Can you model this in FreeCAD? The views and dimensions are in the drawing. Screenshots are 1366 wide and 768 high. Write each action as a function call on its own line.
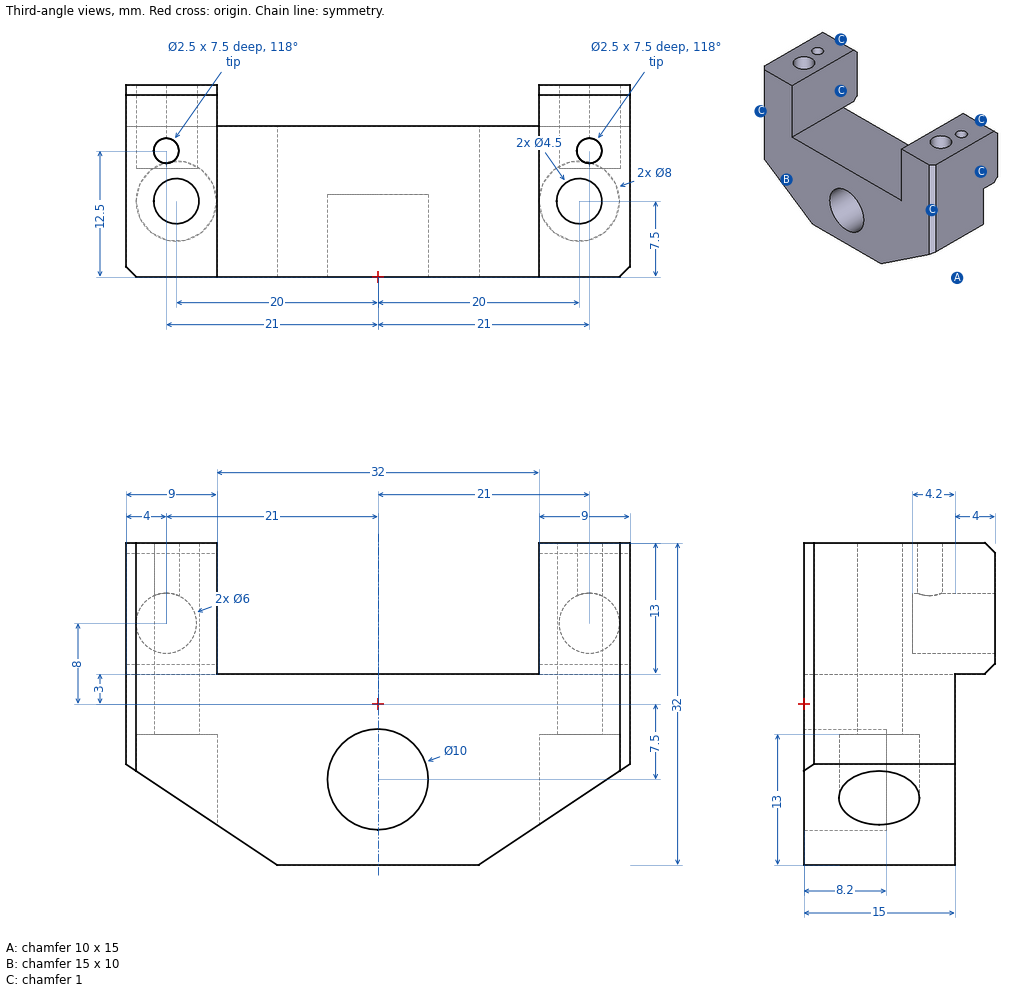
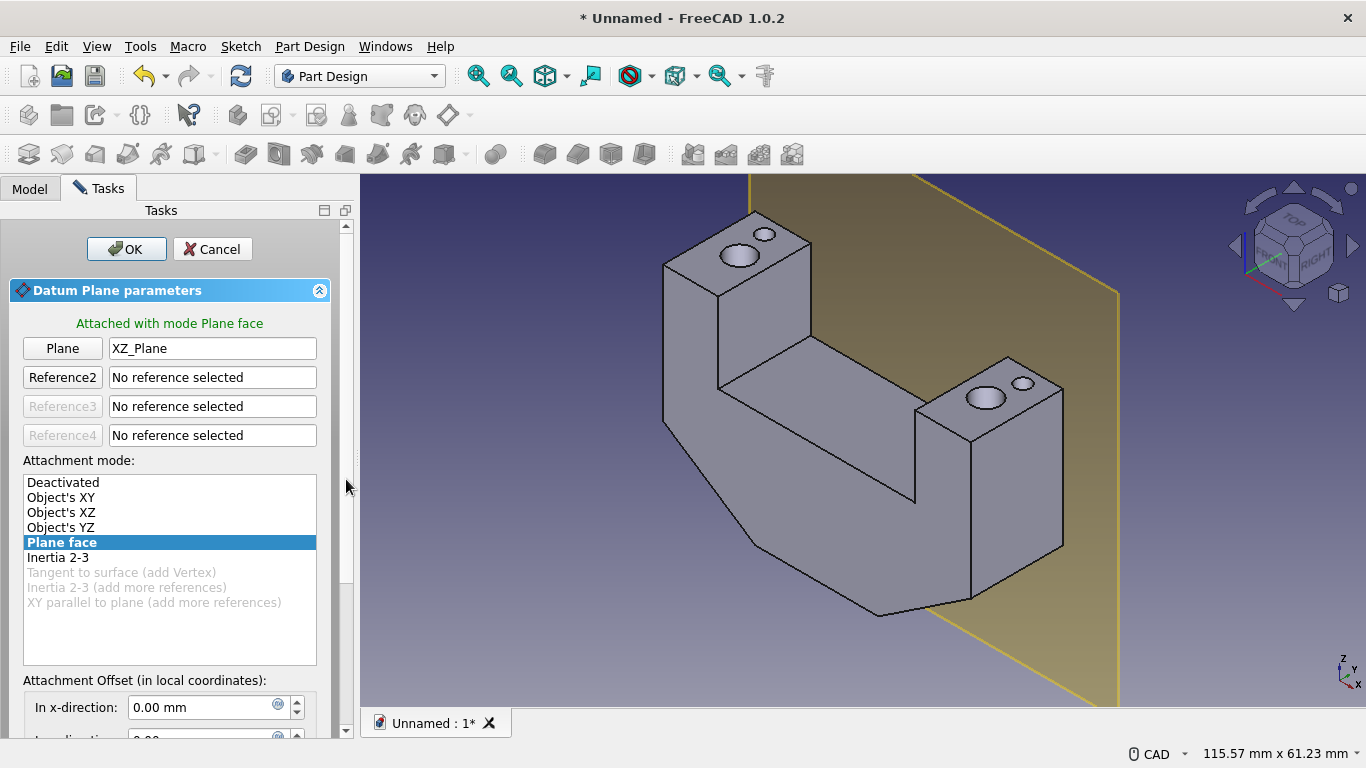
click(127, 249)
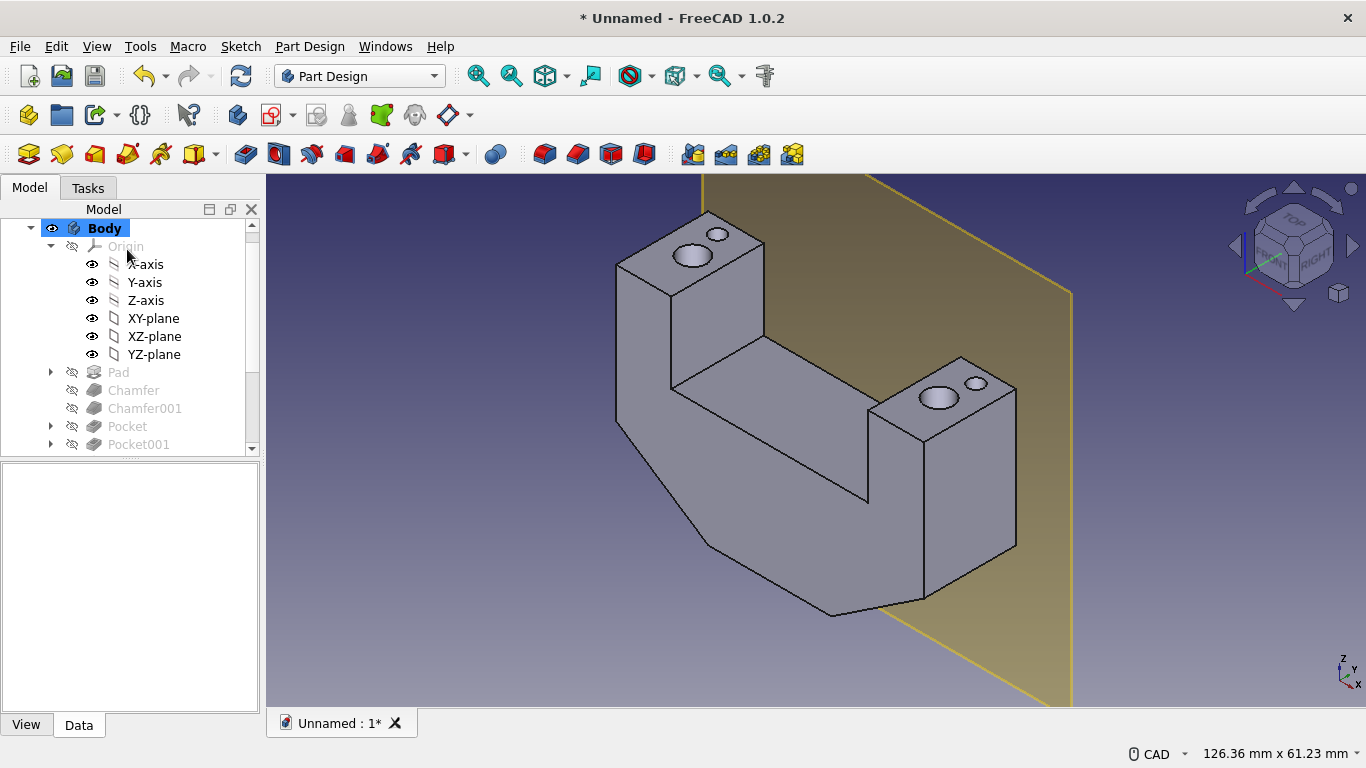
scroll(121, 332, down, 3)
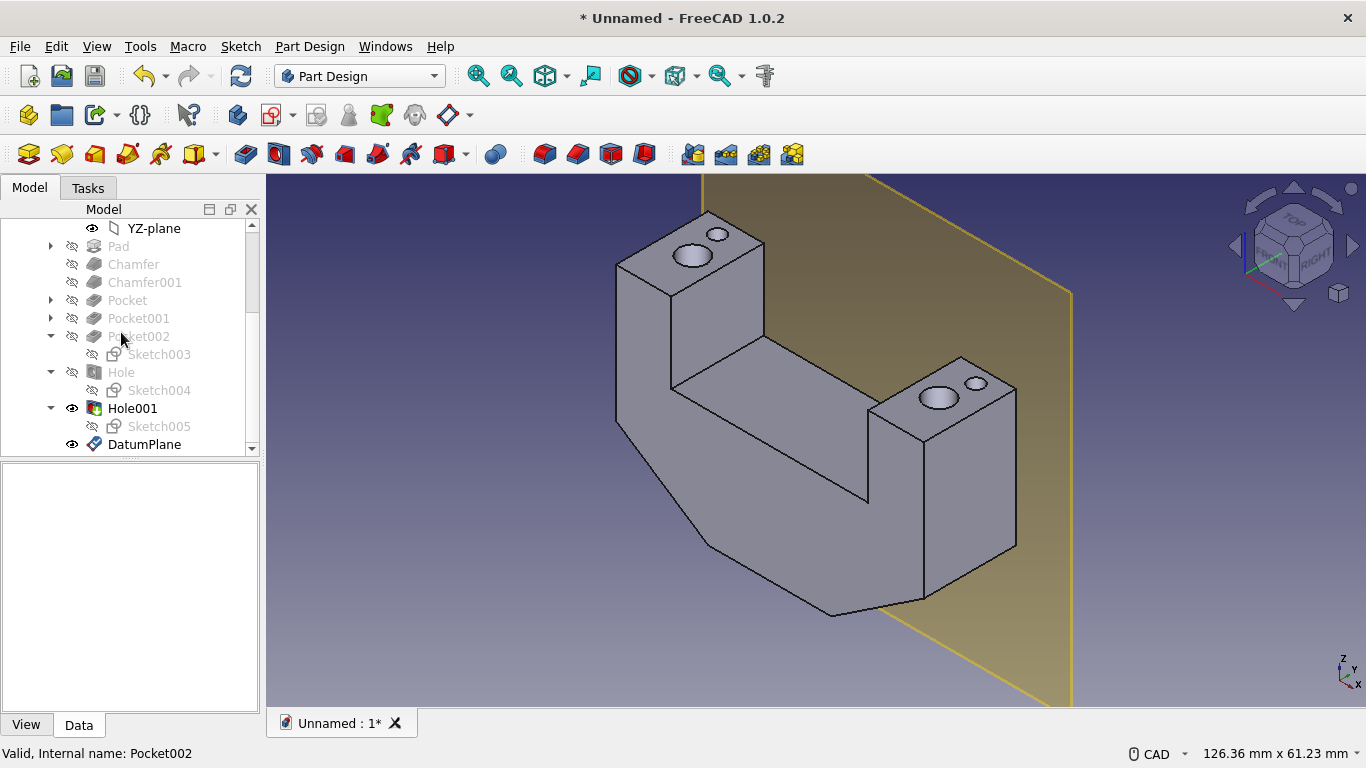
click(117, 444)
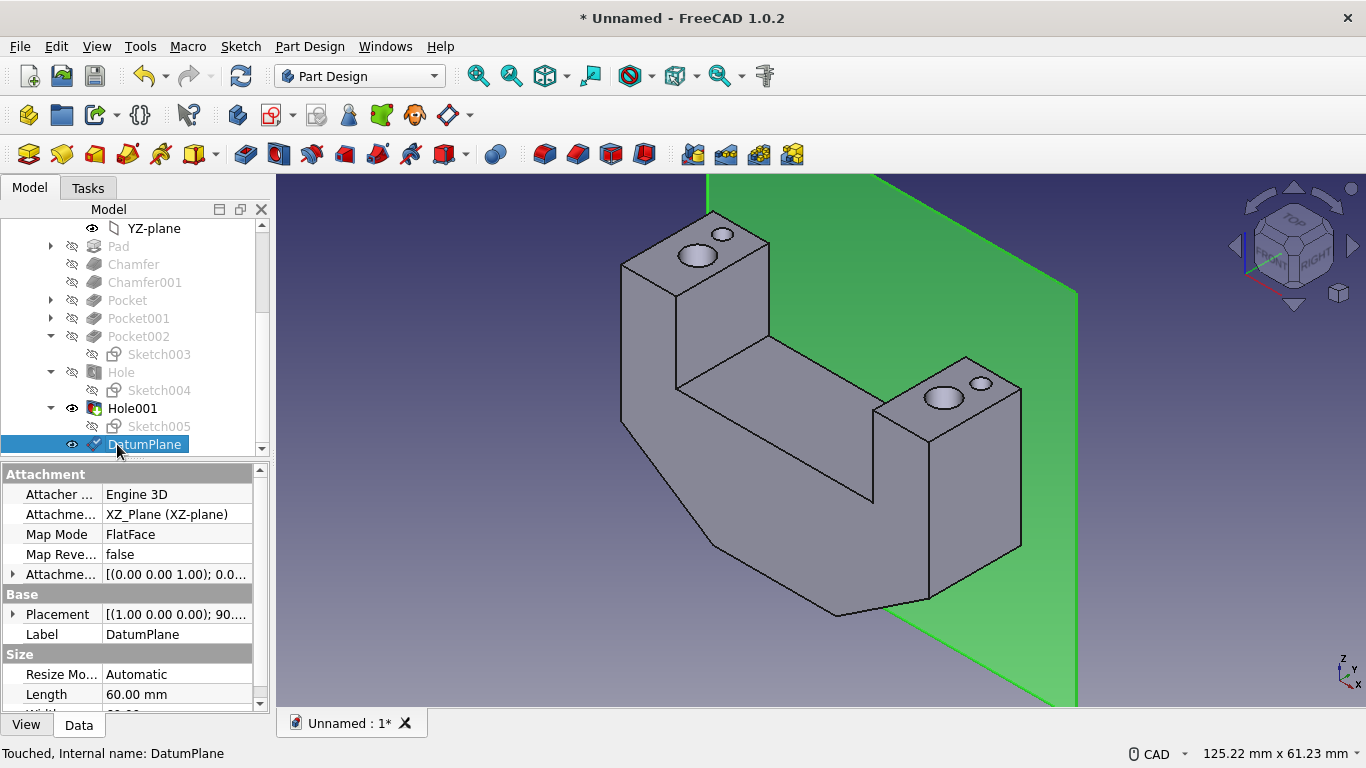
click(270, 116)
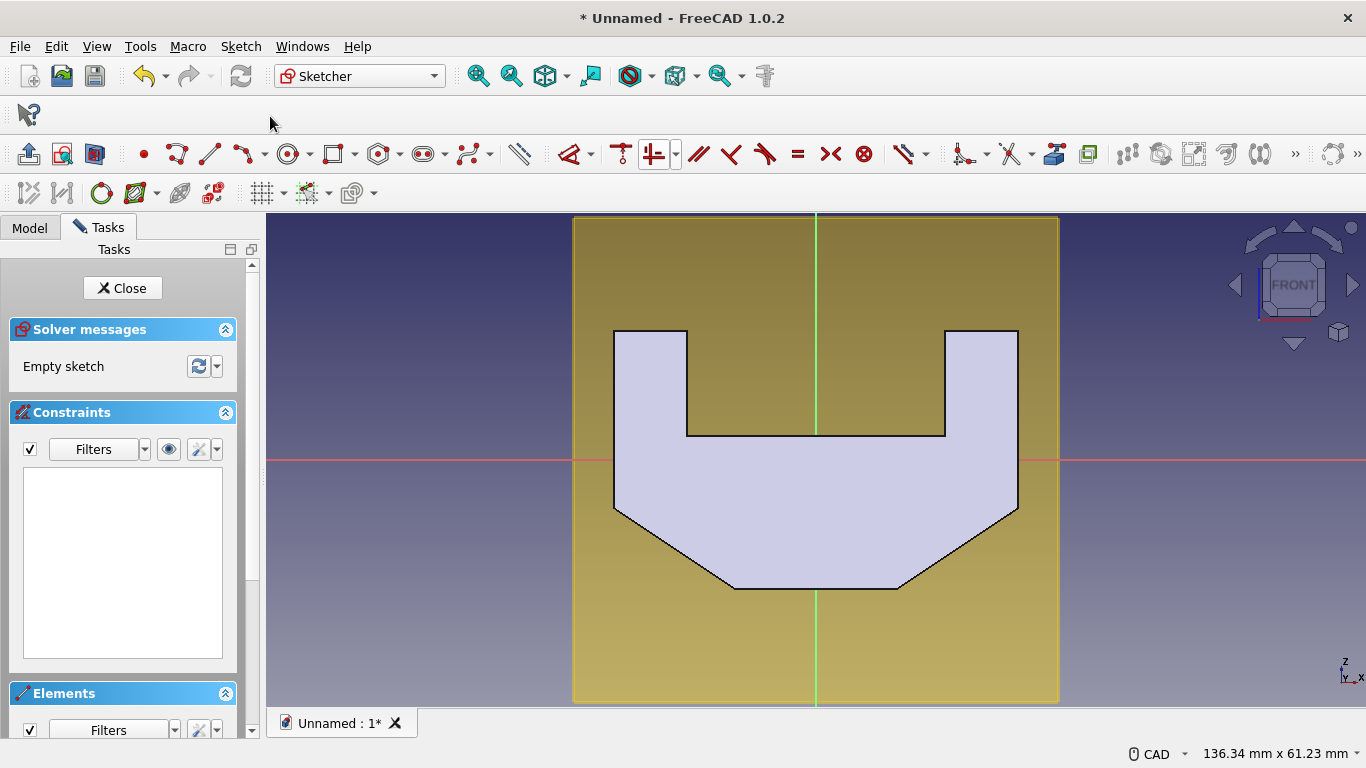
key(q)
key(s)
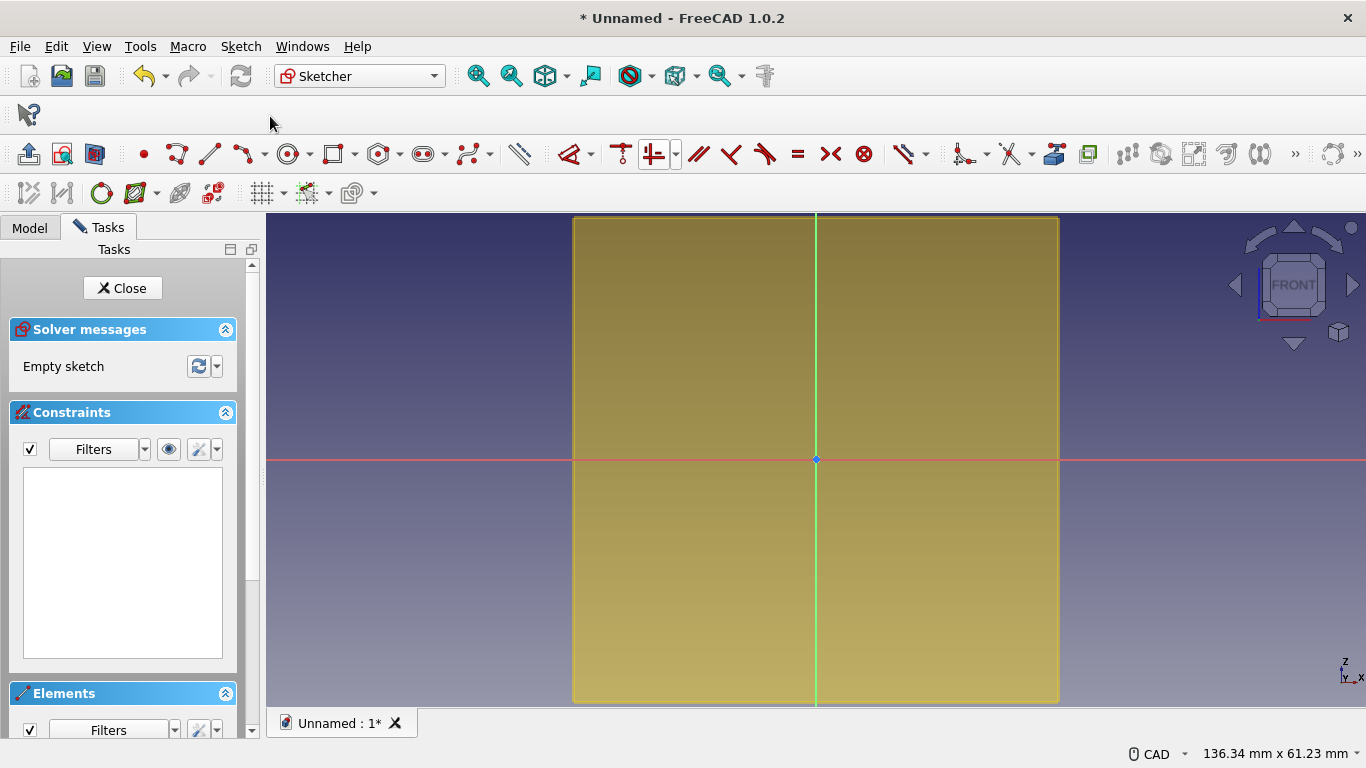
scroll(955, 264, up, 2)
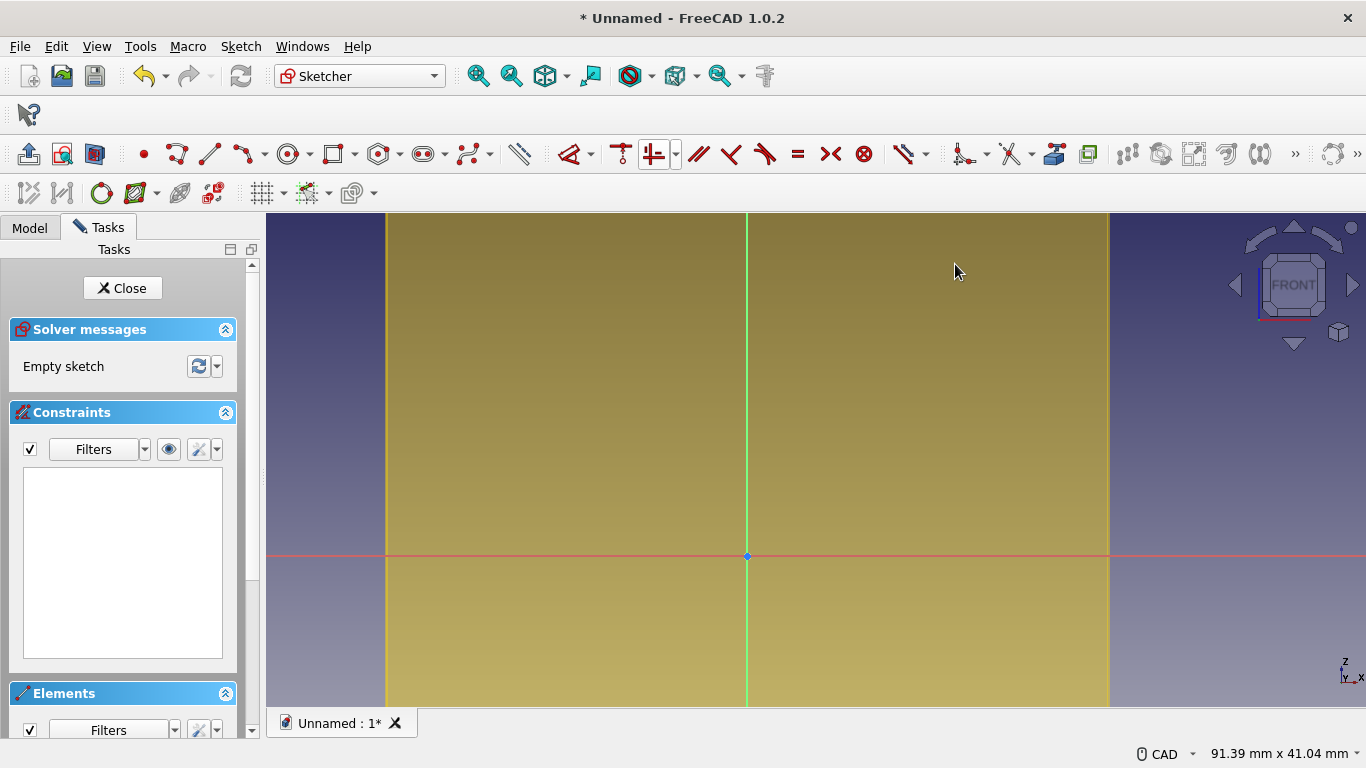
click(332, 154)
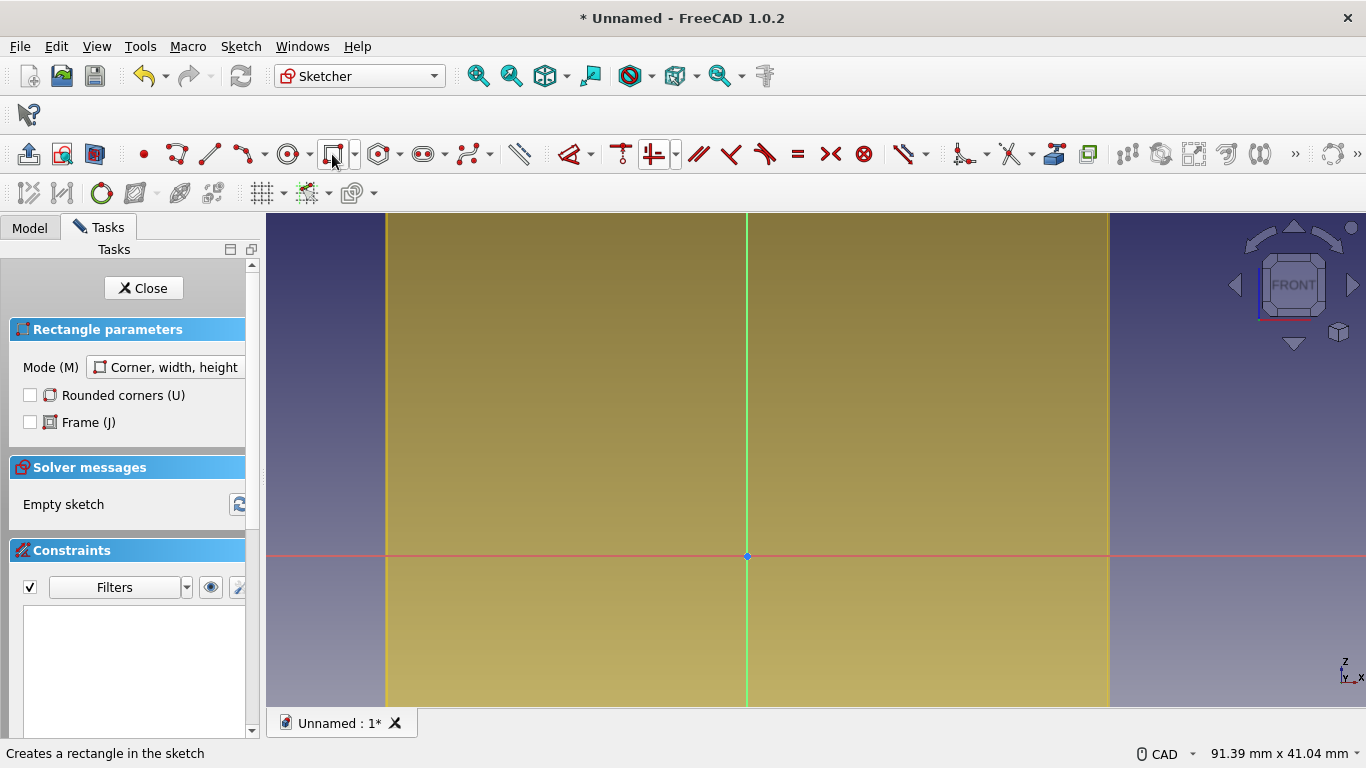
click(446, 364)
move(555, 520)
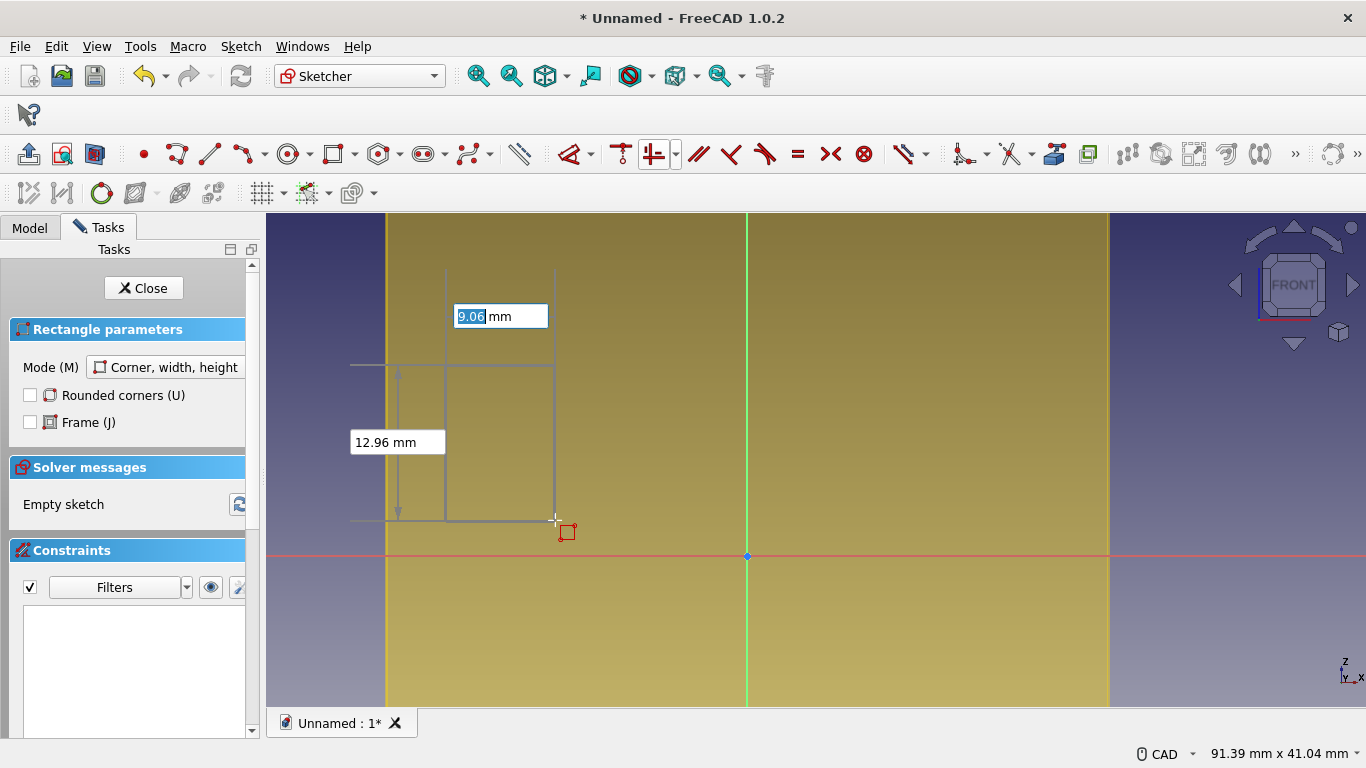
text(9)
key(Tab)
text(13)
key(Return)